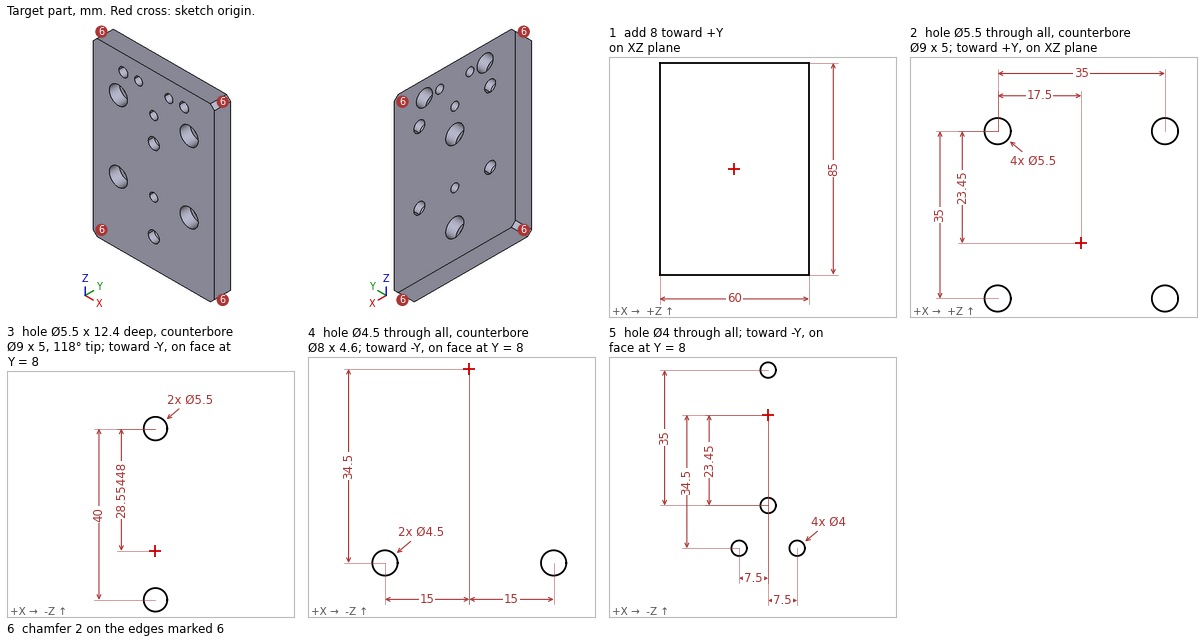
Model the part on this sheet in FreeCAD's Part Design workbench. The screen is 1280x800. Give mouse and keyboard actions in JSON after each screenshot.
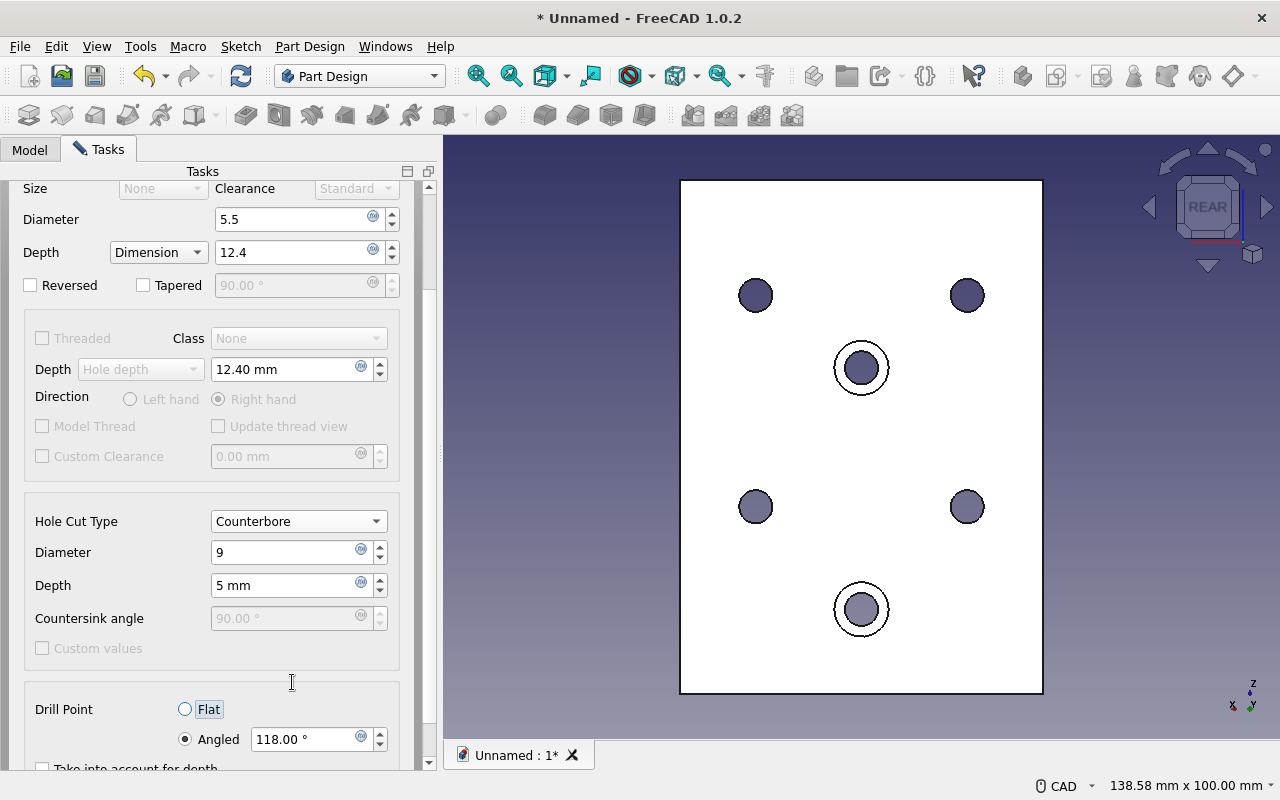
{"action": "scroll", "coordinate": [429, 476], "scroll_direction": "up", "scroll_amount": 3}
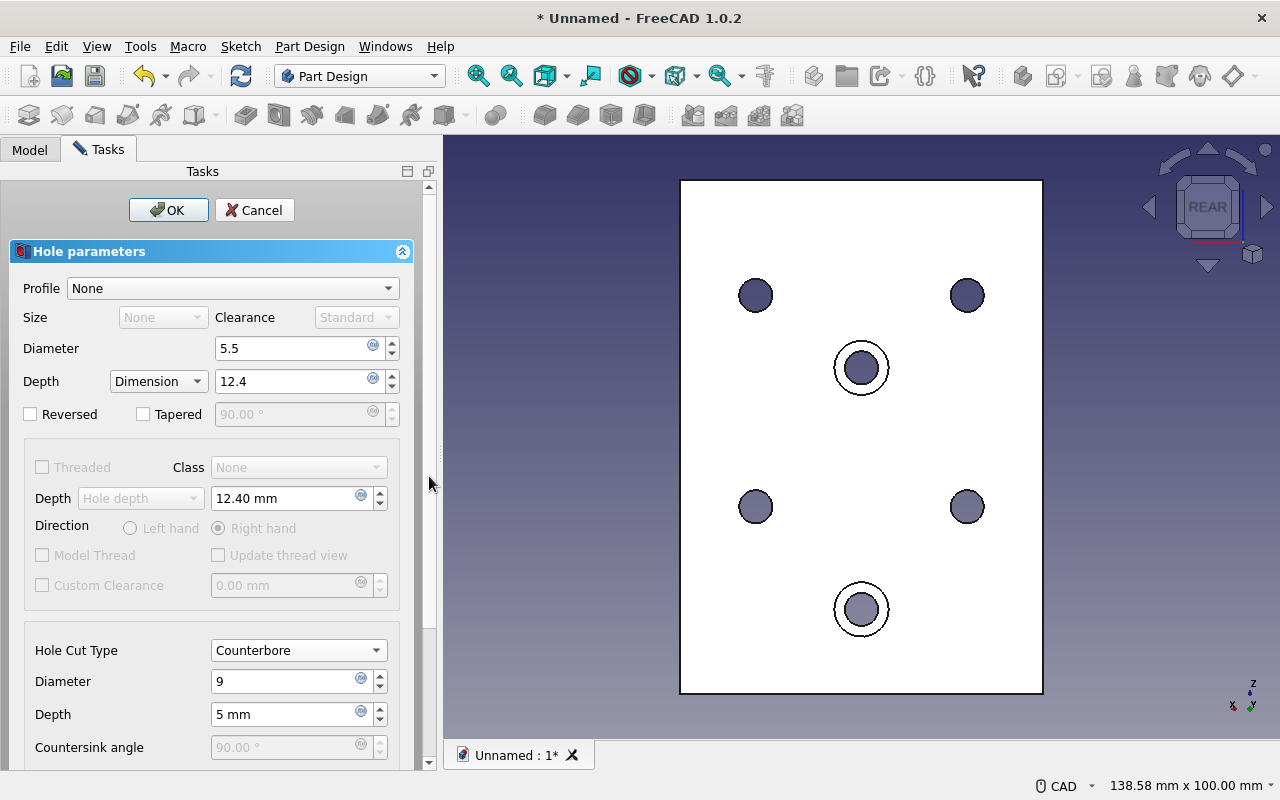
{"action": "left_click", "coordinate": [169, 210]}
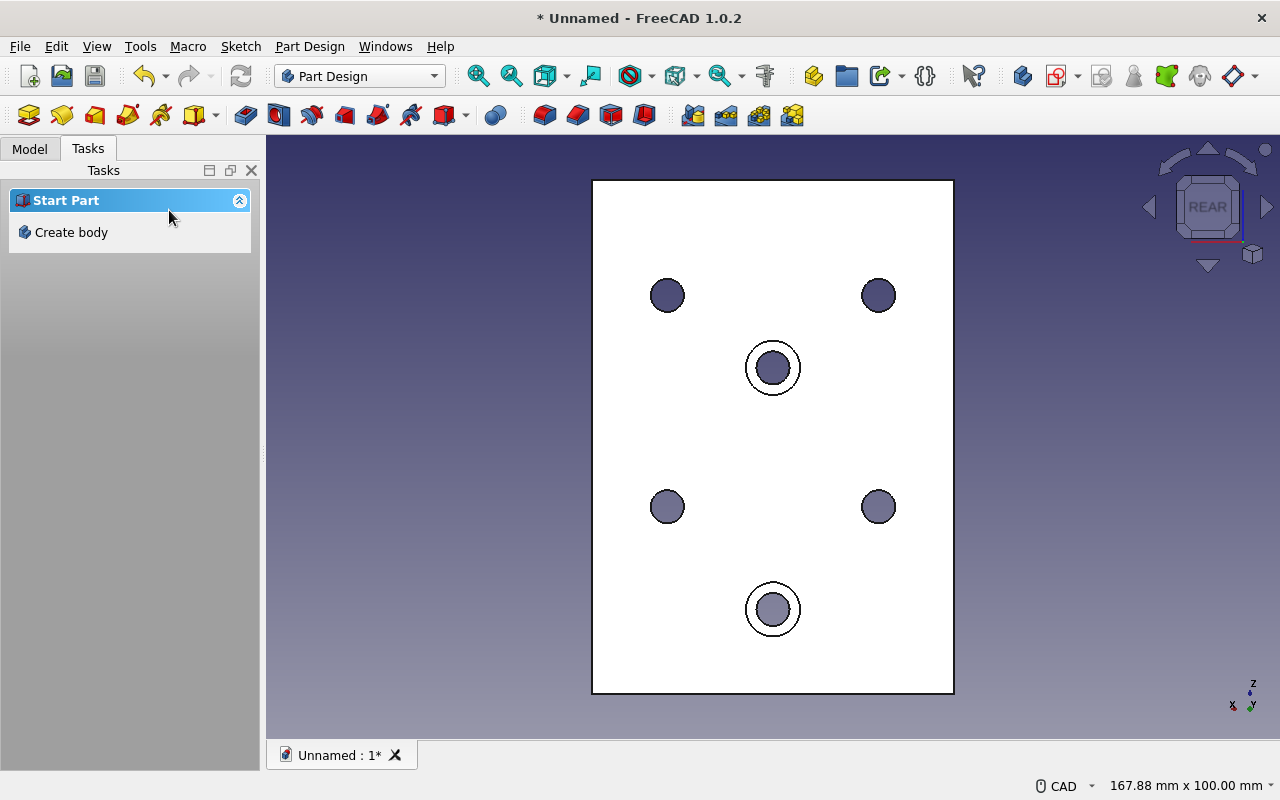
{"action": "left_click", "coordinate": [773, 509]}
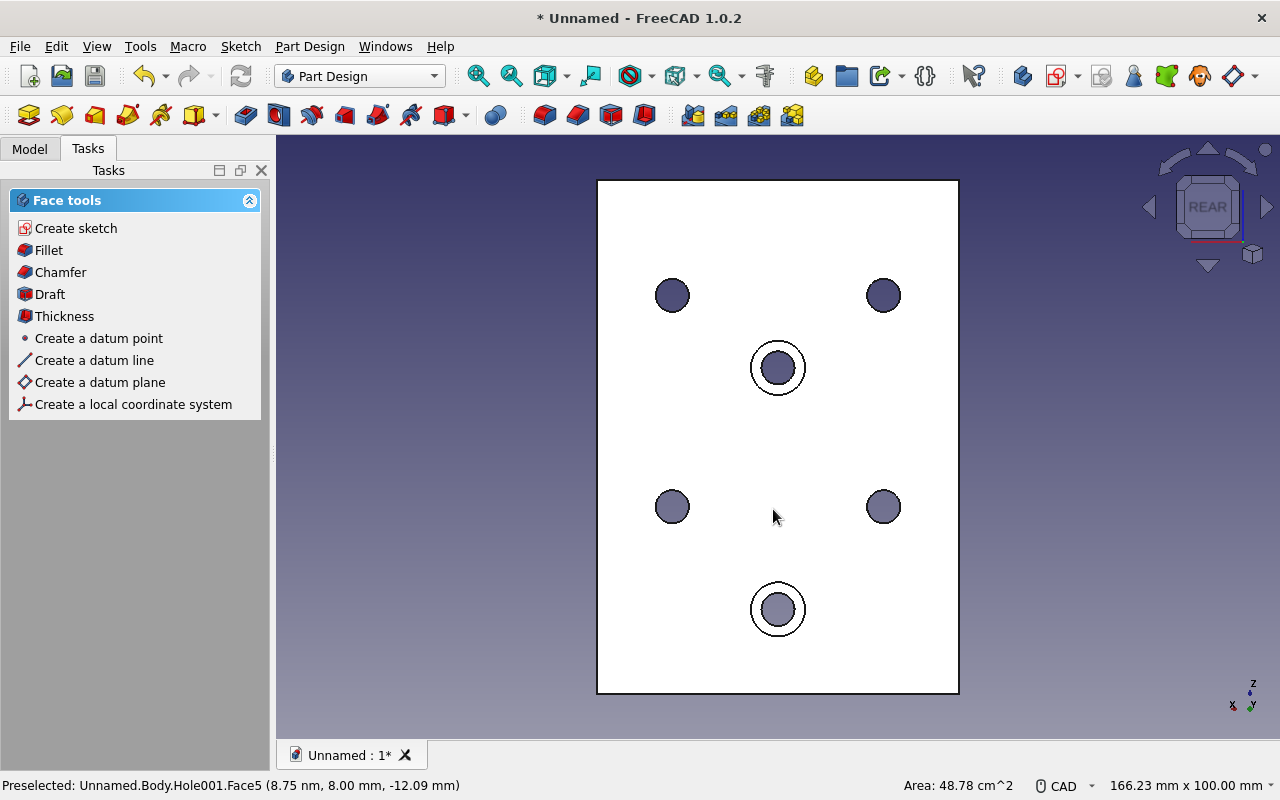
{"action": "left_click", "coordinate": [1056, 76]}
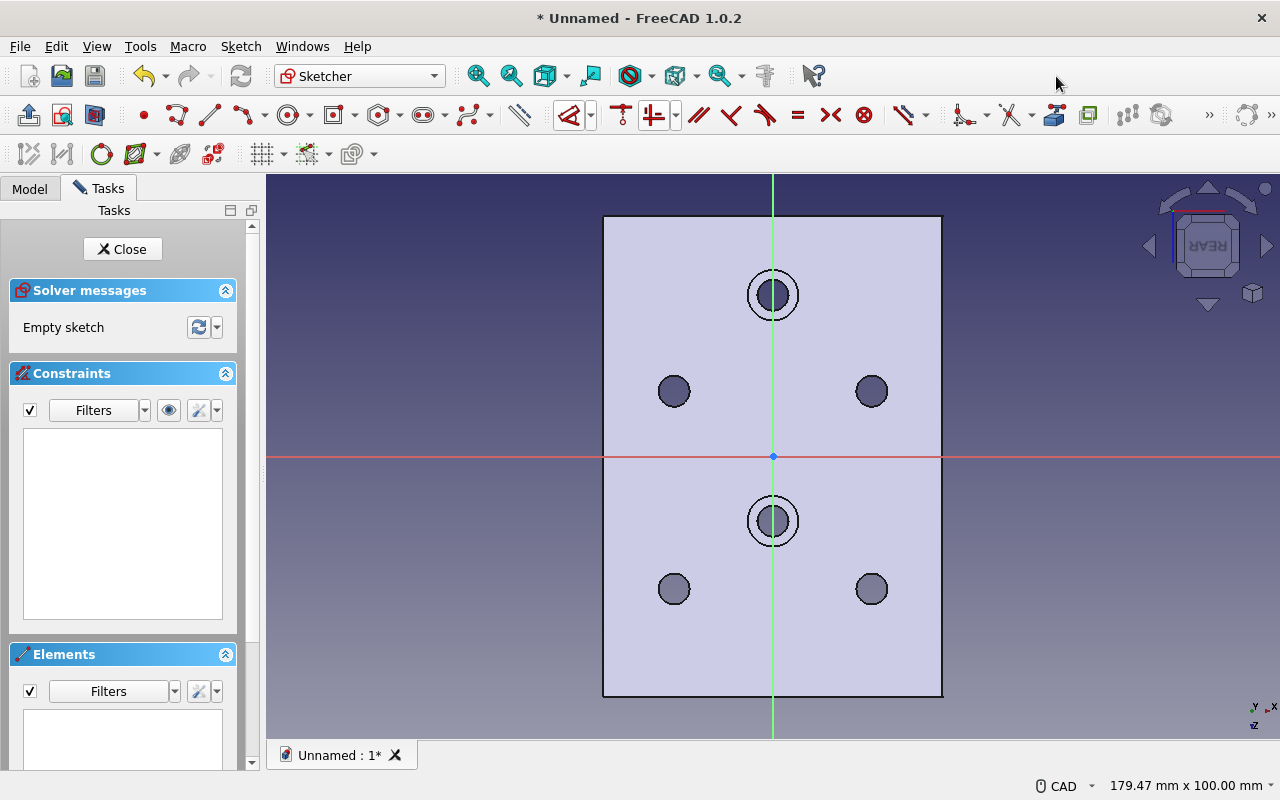
{"action": "scroll", "coordinate": [856, 687], "scroll_direction": "up", "scroll_amount": 3}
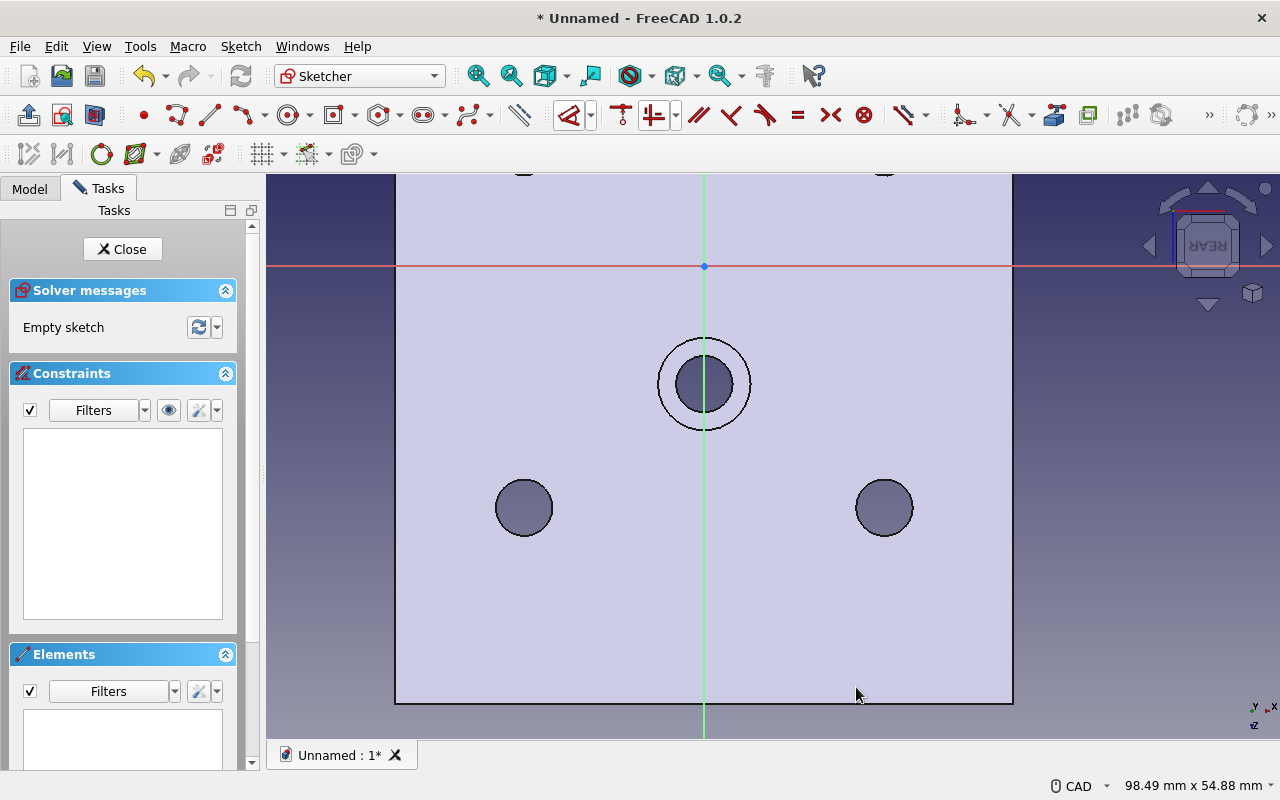
{"action": "key", "text": "g c"}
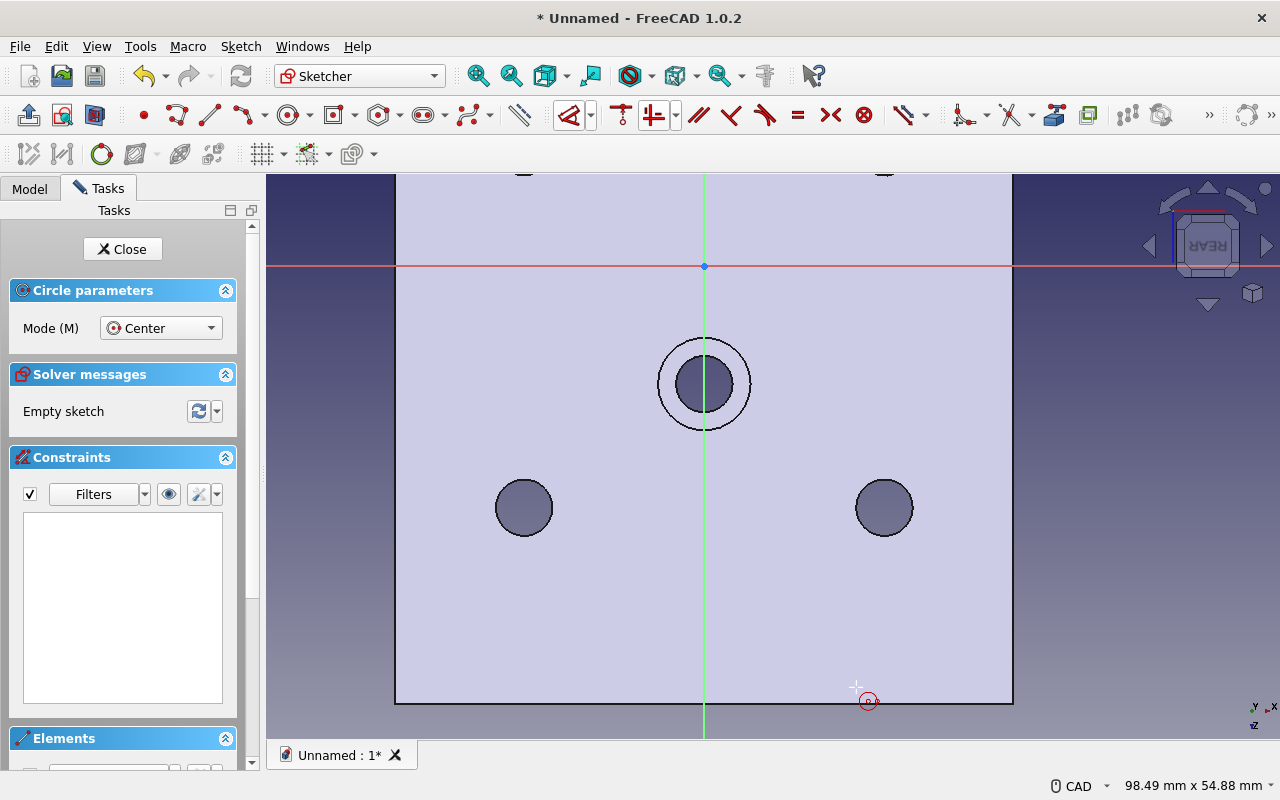
{"action": "left_click", "coordinate": [550, 621]}
{"action": "left_click", "coordinate": [566, 605]}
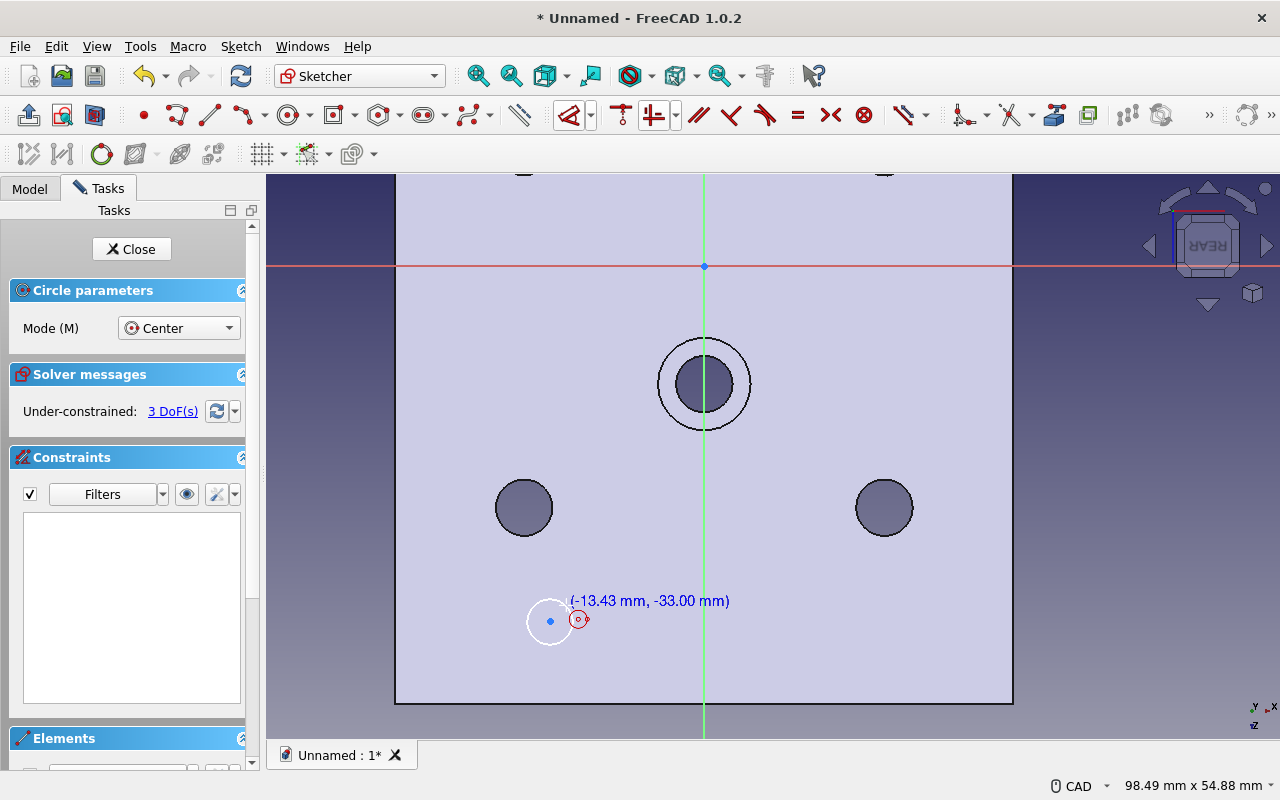
{"action": "left_click", "coordinate": [859, 621]}
{"action": "left_click", "coordinate": [875, 605]}
{"action": "key", "text": "Escape"}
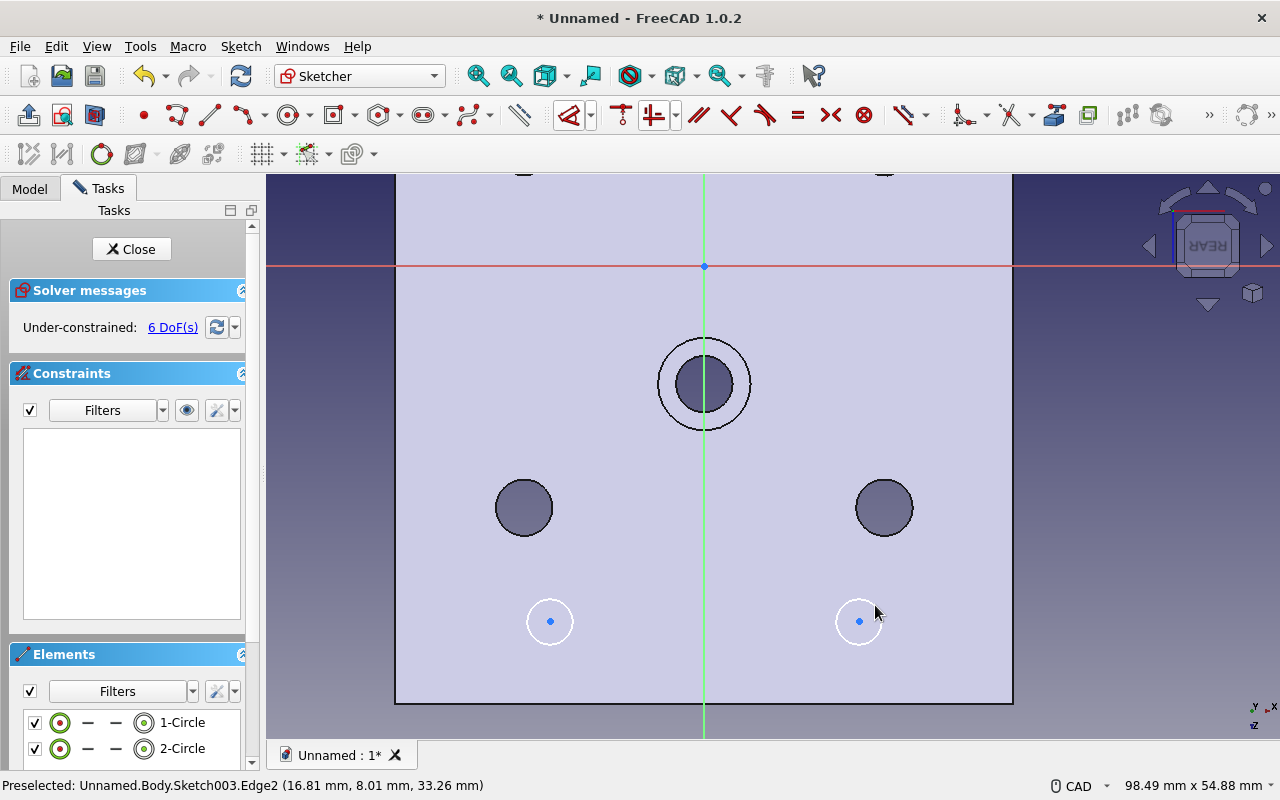
{"action": "left_click", "coordinate": [566, 606]}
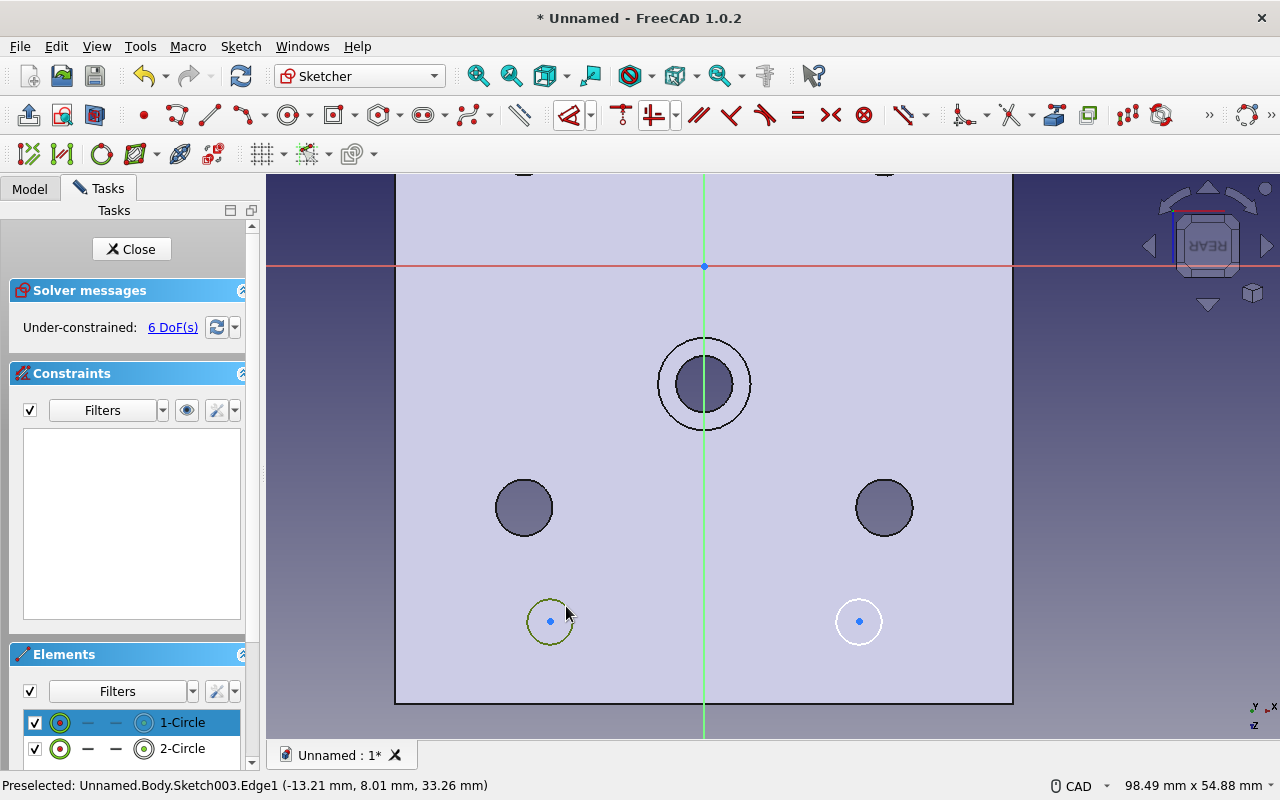
{"action": "left_click", "coordinate": [875, 606]}